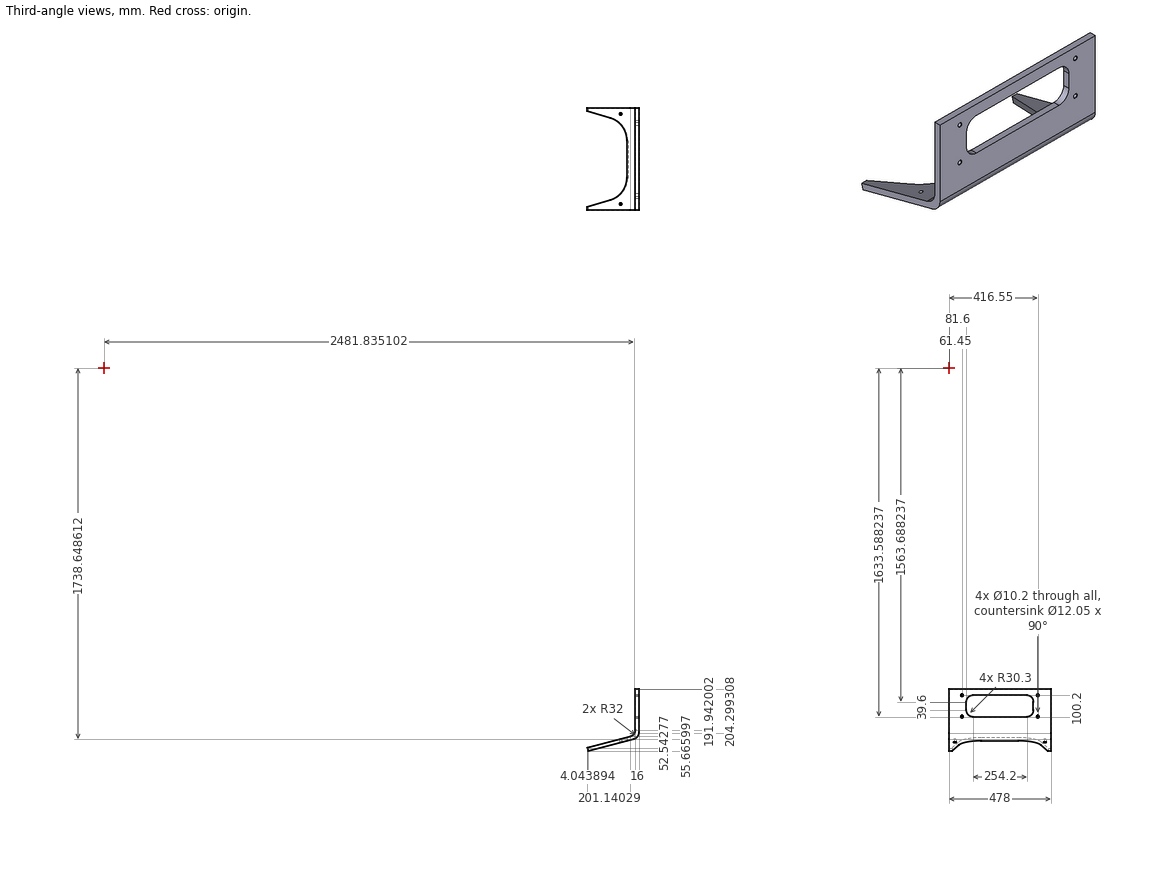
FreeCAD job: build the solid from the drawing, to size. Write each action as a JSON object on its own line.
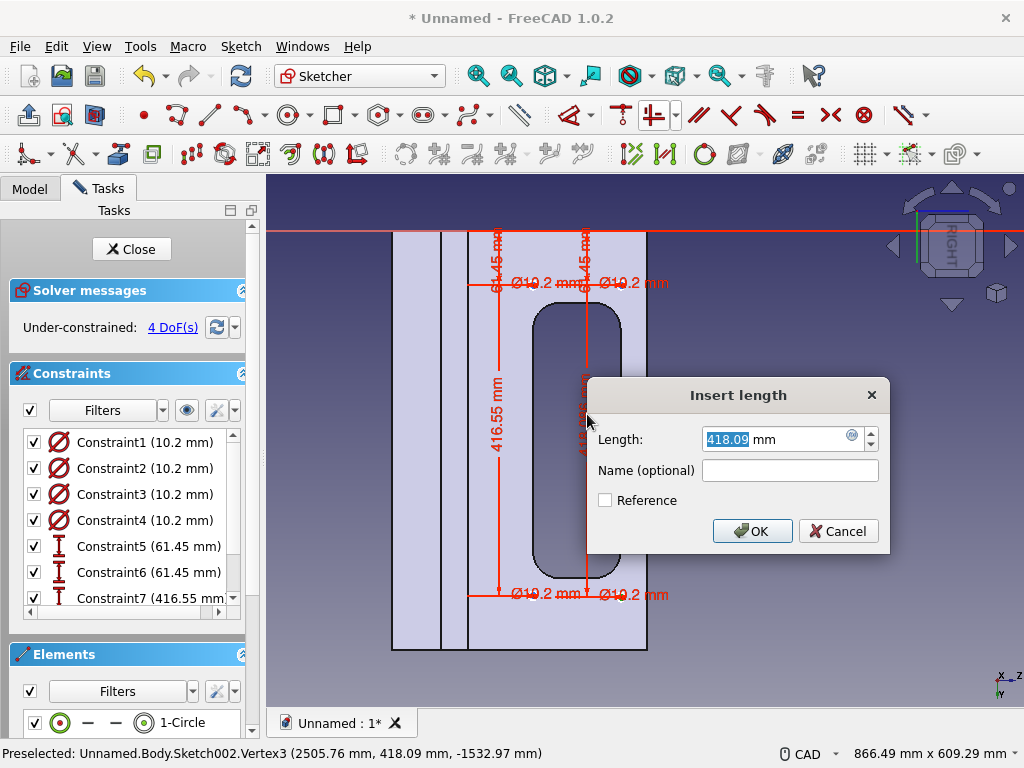
{"action": "type", "text": "416.55"}
{"action": "key", "text": "Return"}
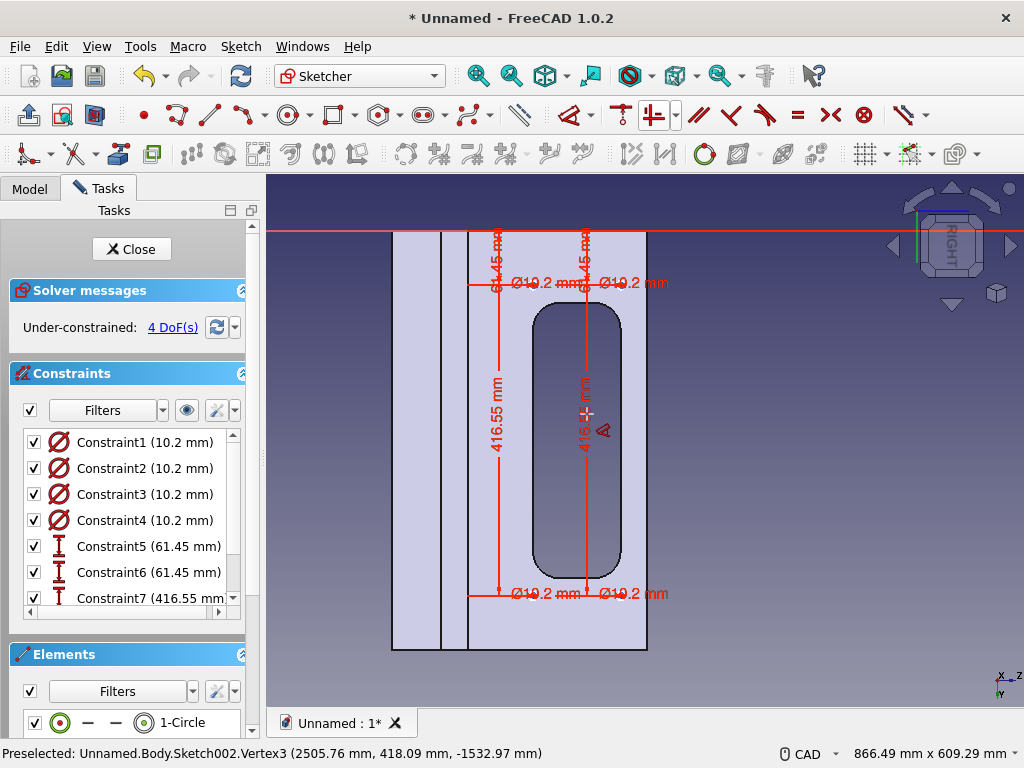
{"action": "left_click", "coordinate": [533, 596]}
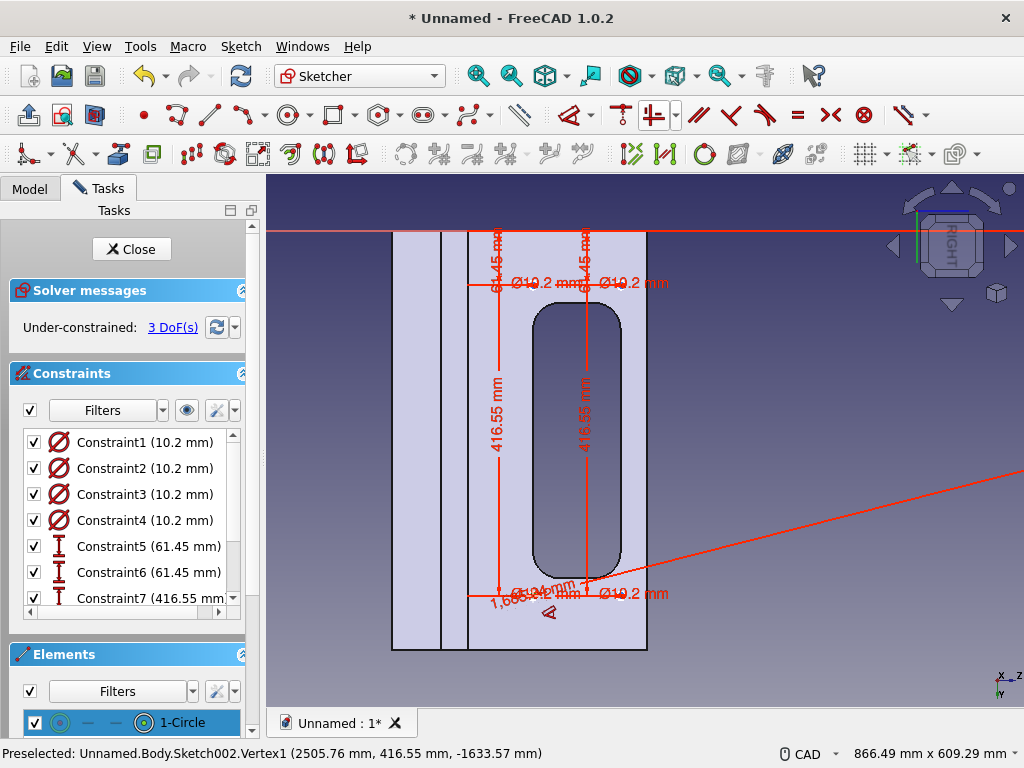
{"action": "left_click", "coordinate": [621, 285]}
{"action": "left_click", "coordinate": [577, 630]}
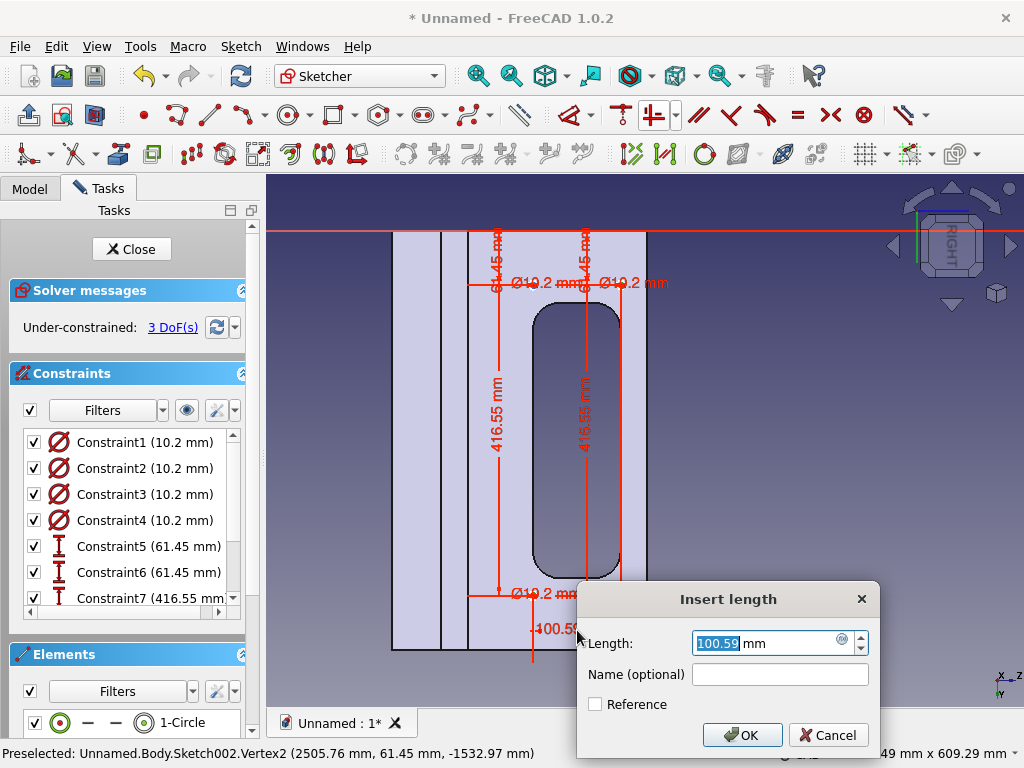
{"action": "type", "text": "100.2"}
{"action": "key", "text": "Return"}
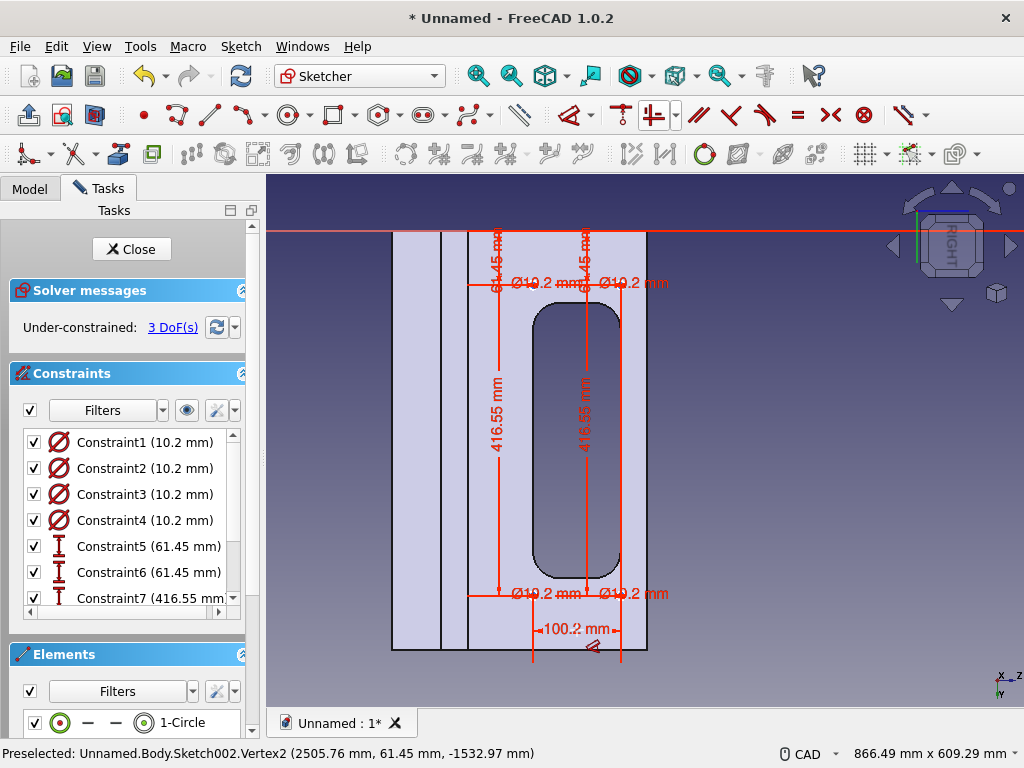
{"action": "left_click", "coordinate": [533, 596]}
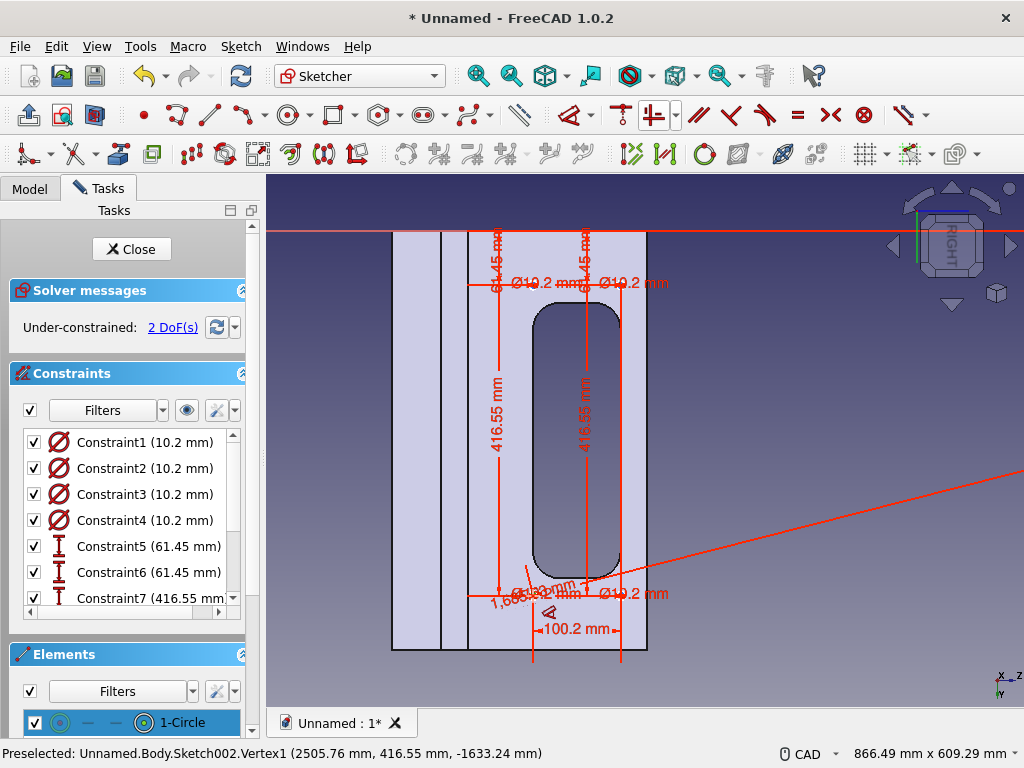
{"action": "left_click", "coordinate": [621, 596]}
{"action": "left_click", "coordinate": [577, 562]}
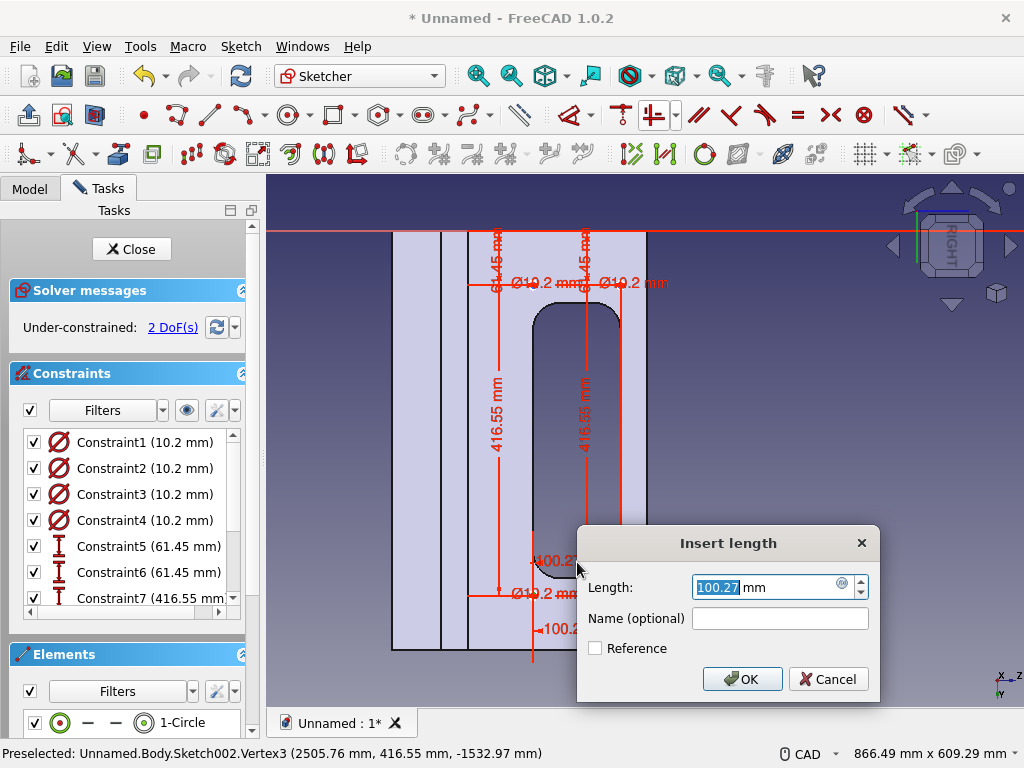
{"action": "type", "text": "100.2"}
{"action": "key", "text": "Return"}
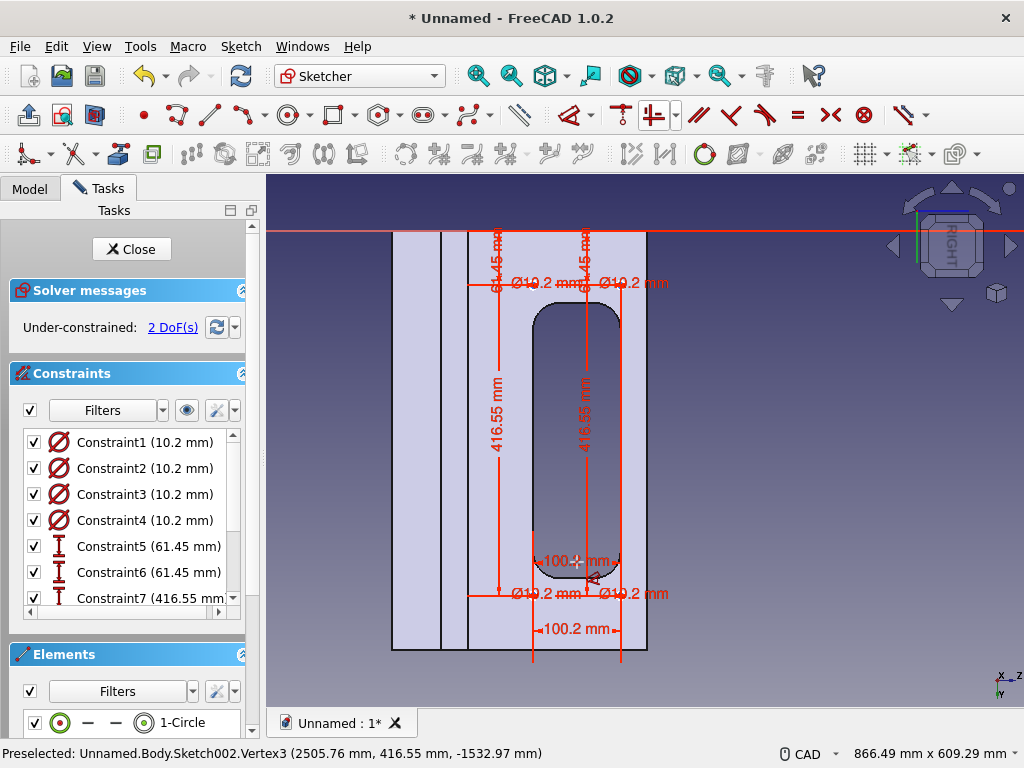
{"action": "left_click", "coordinate": [621, 285]}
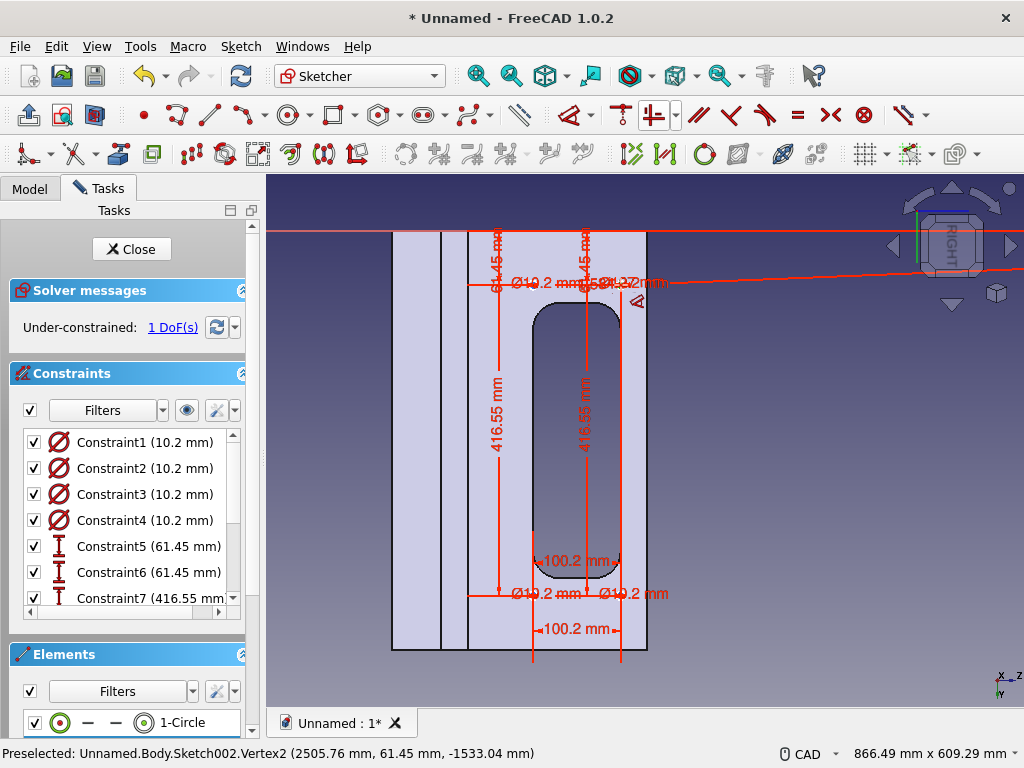
{"action": "left_click", "coordinate": [533, 285]}
{"action": "left_click", "coordinate": [577, 319]}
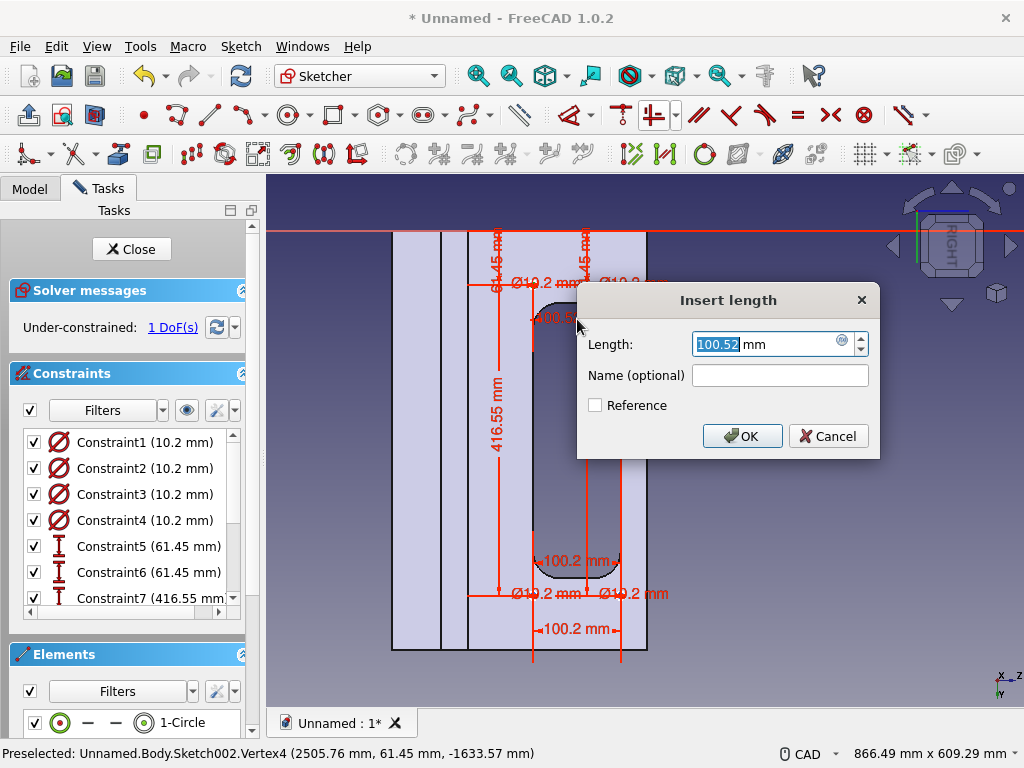
{"action": "type", "text": "100.2"}
{"action": "key", "text": "Return"}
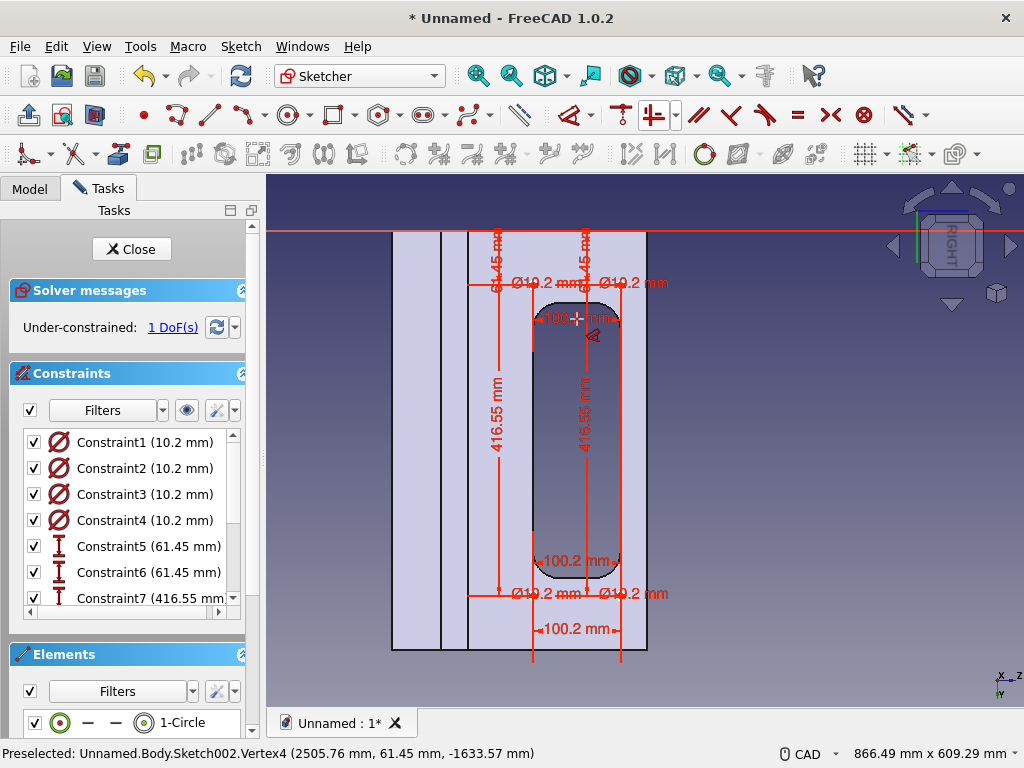
{"action": "left_click", "coordinate": [533, 596]}
{"action": "left_click", "coordinate": [696, 630]}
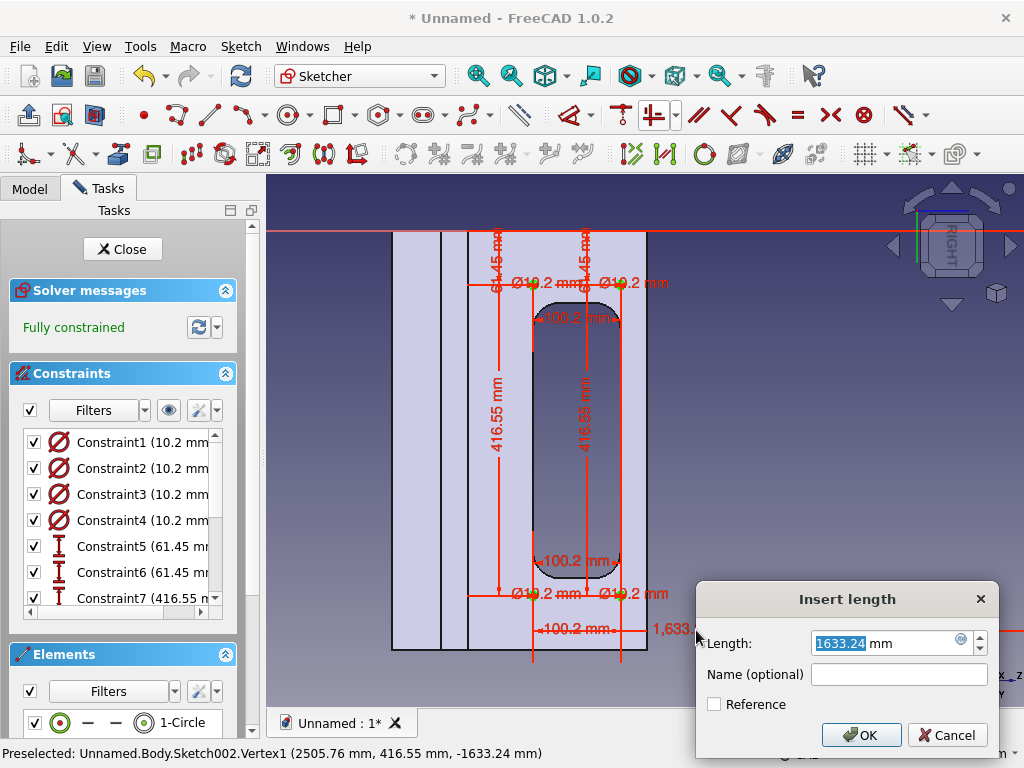
{"action": "type", "text": "1633.588237"}
{"action": "key", "text": "Return"}
{"action": "key", "text": "Escape"}